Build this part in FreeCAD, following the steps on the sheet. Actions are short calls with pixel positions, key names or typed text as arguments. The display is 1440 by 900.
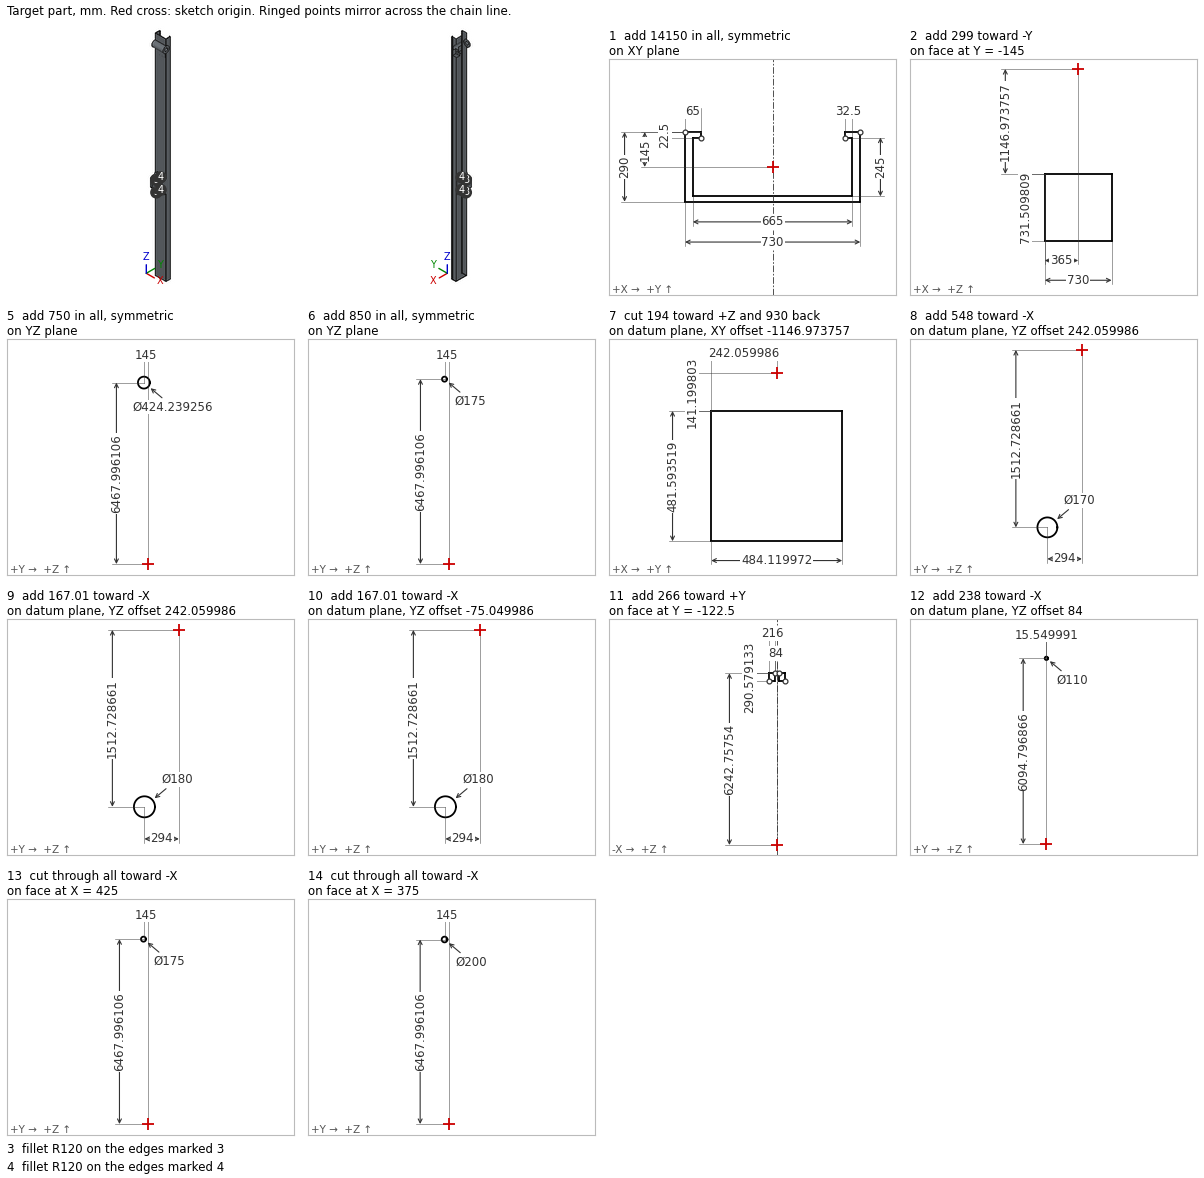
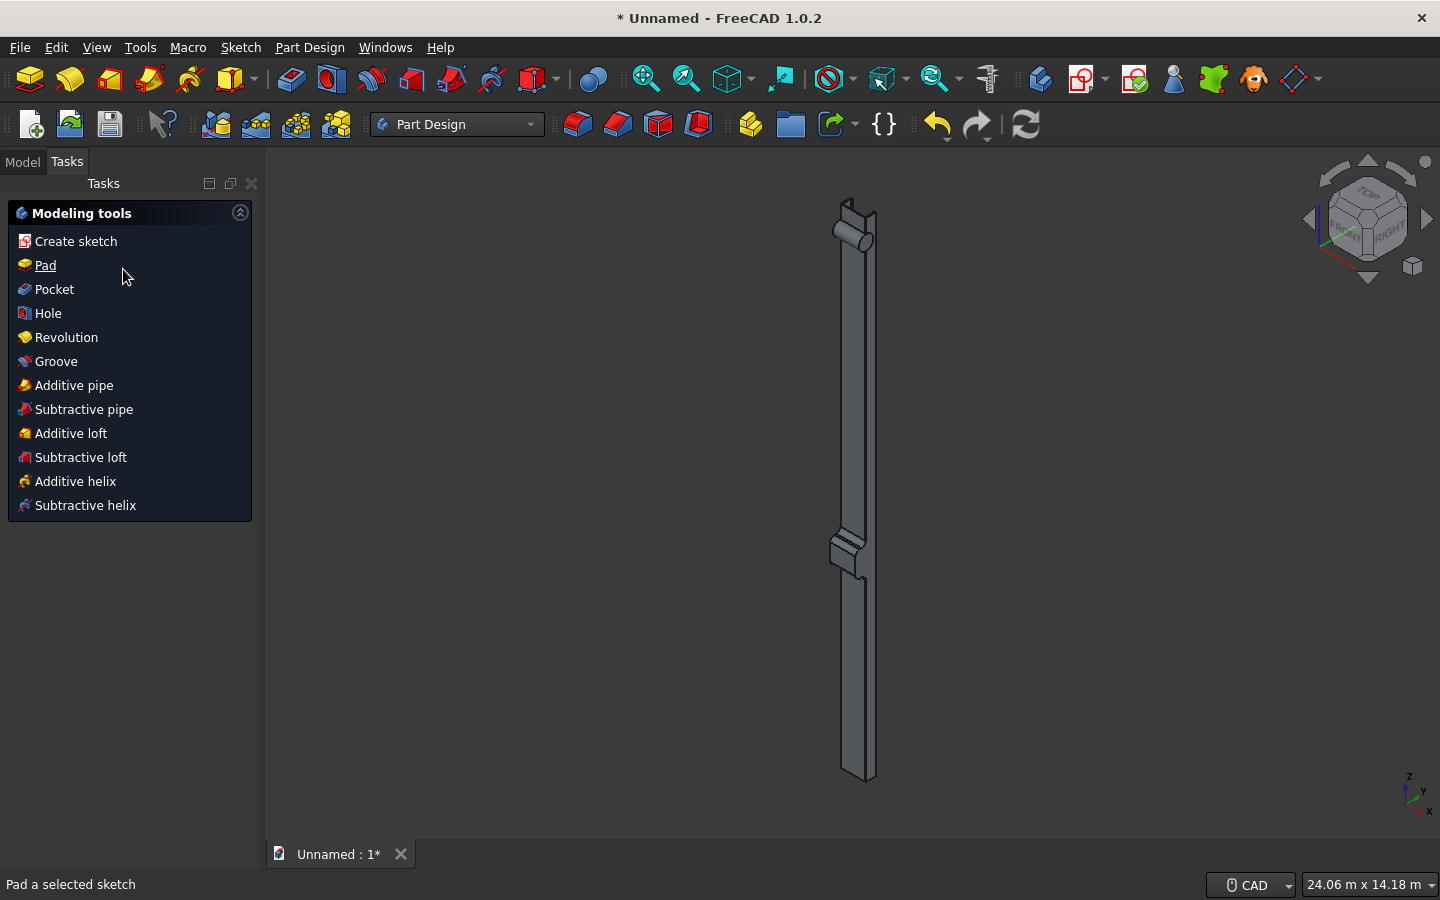
click(30, 80)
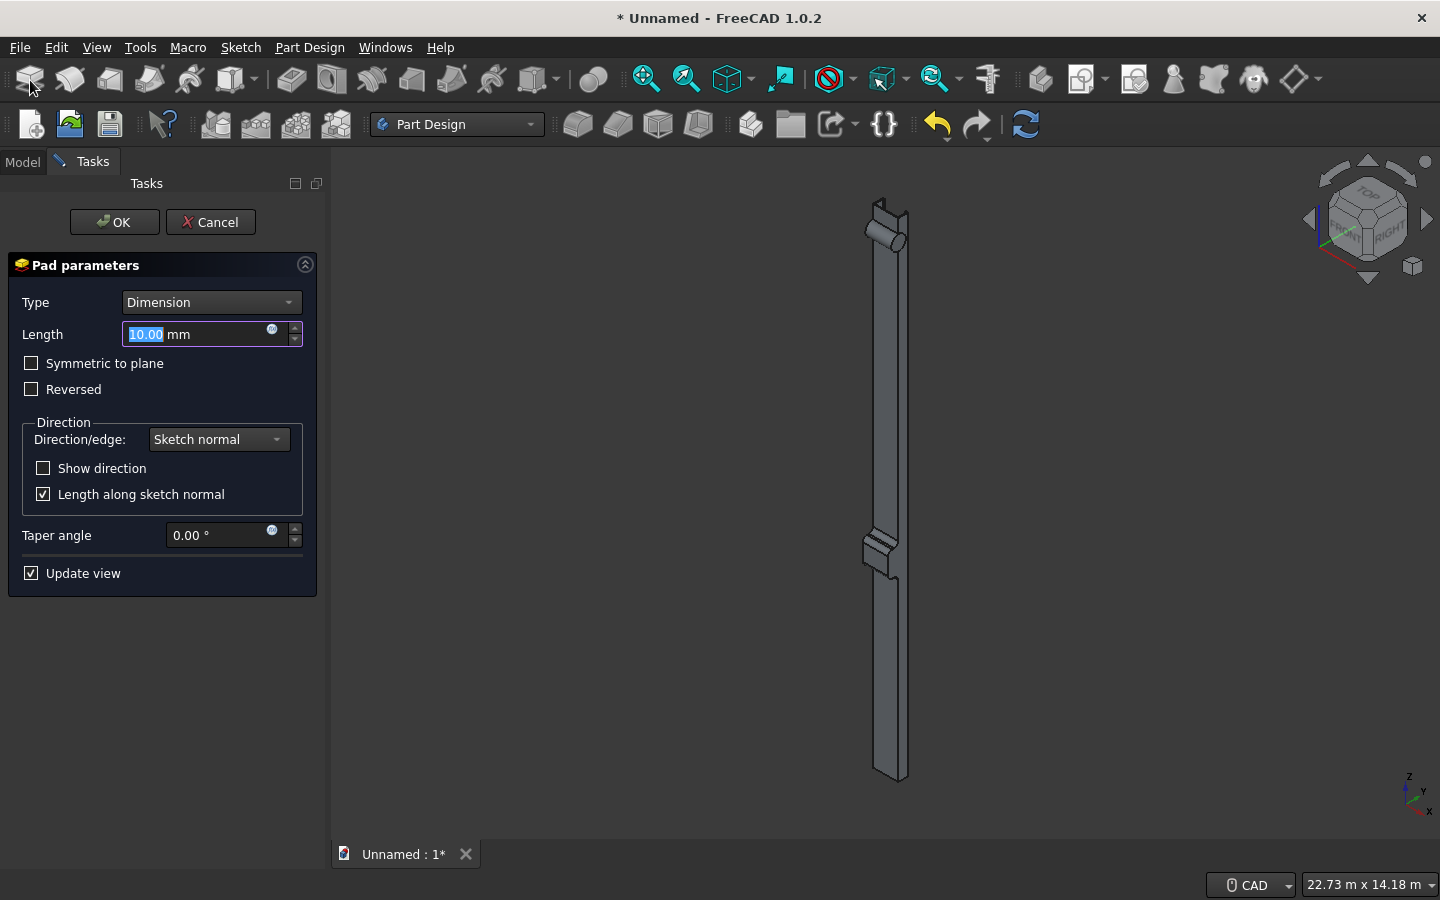
text(850)
key(Tab)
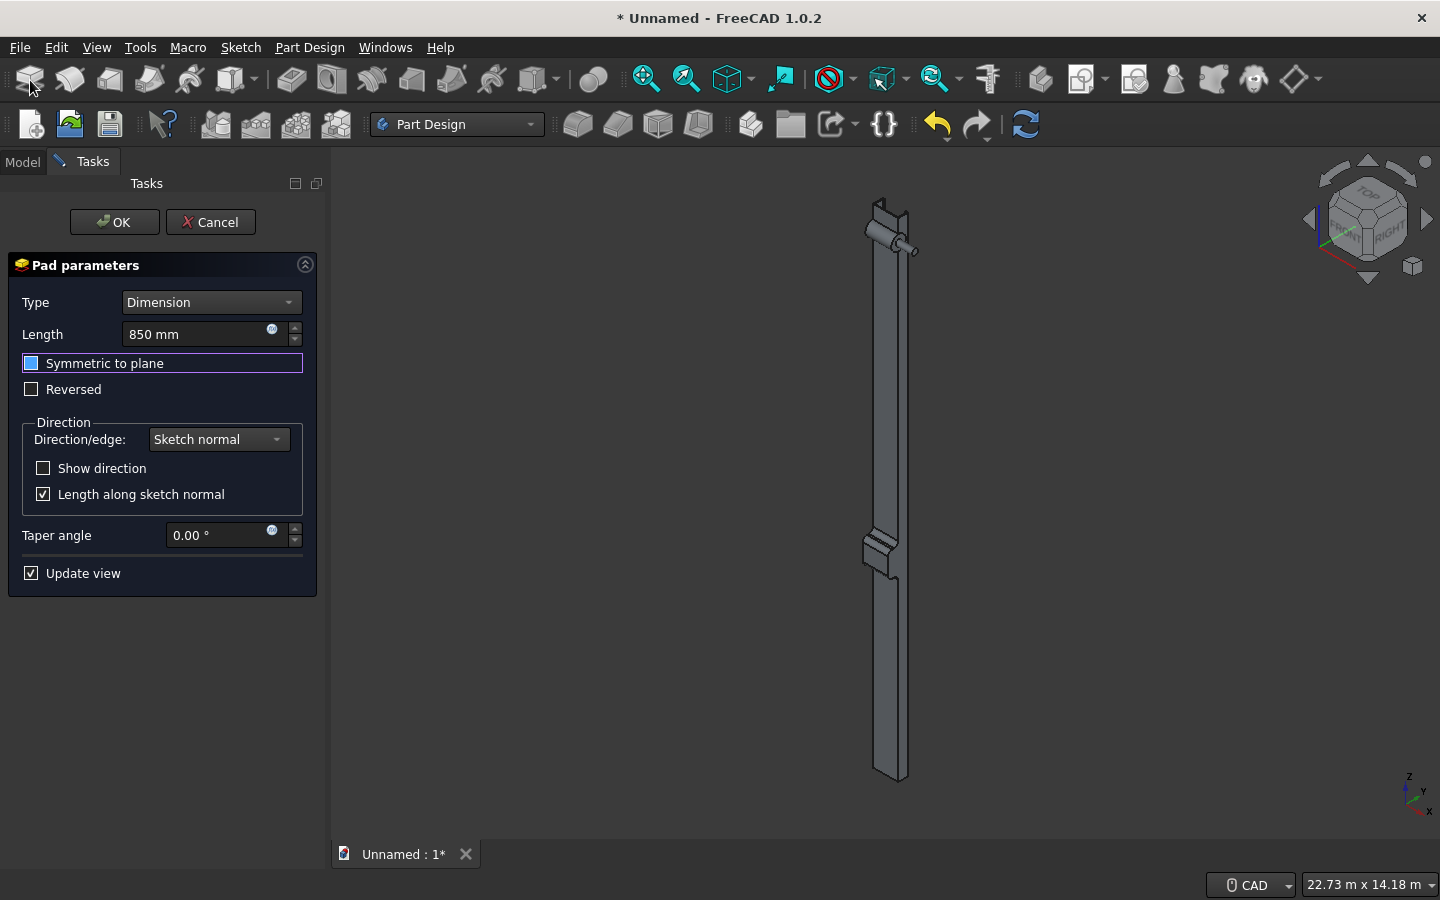
click(30, 363)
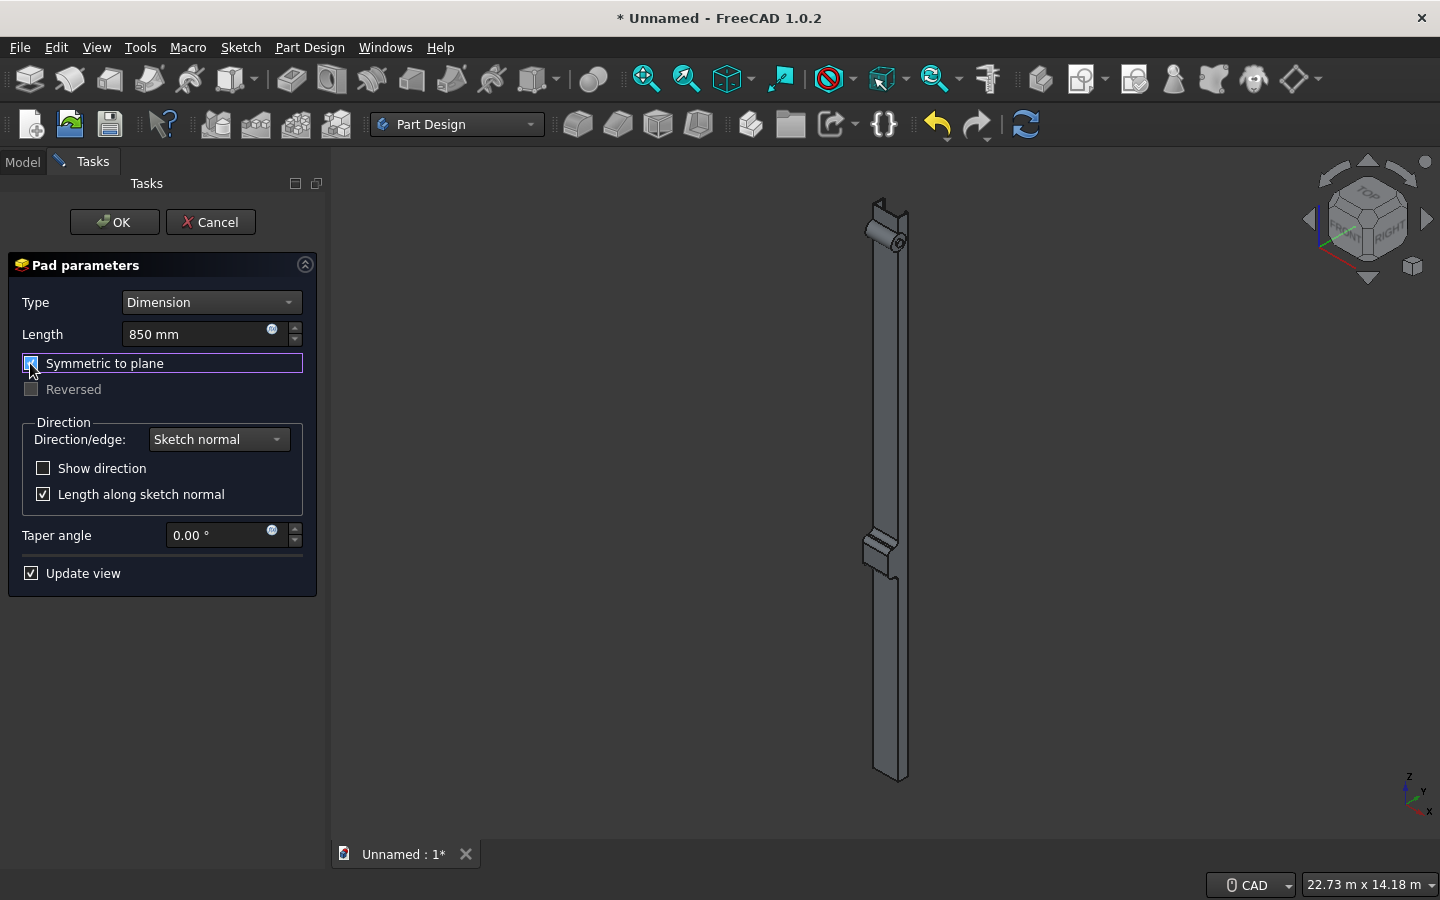
click(115, 222)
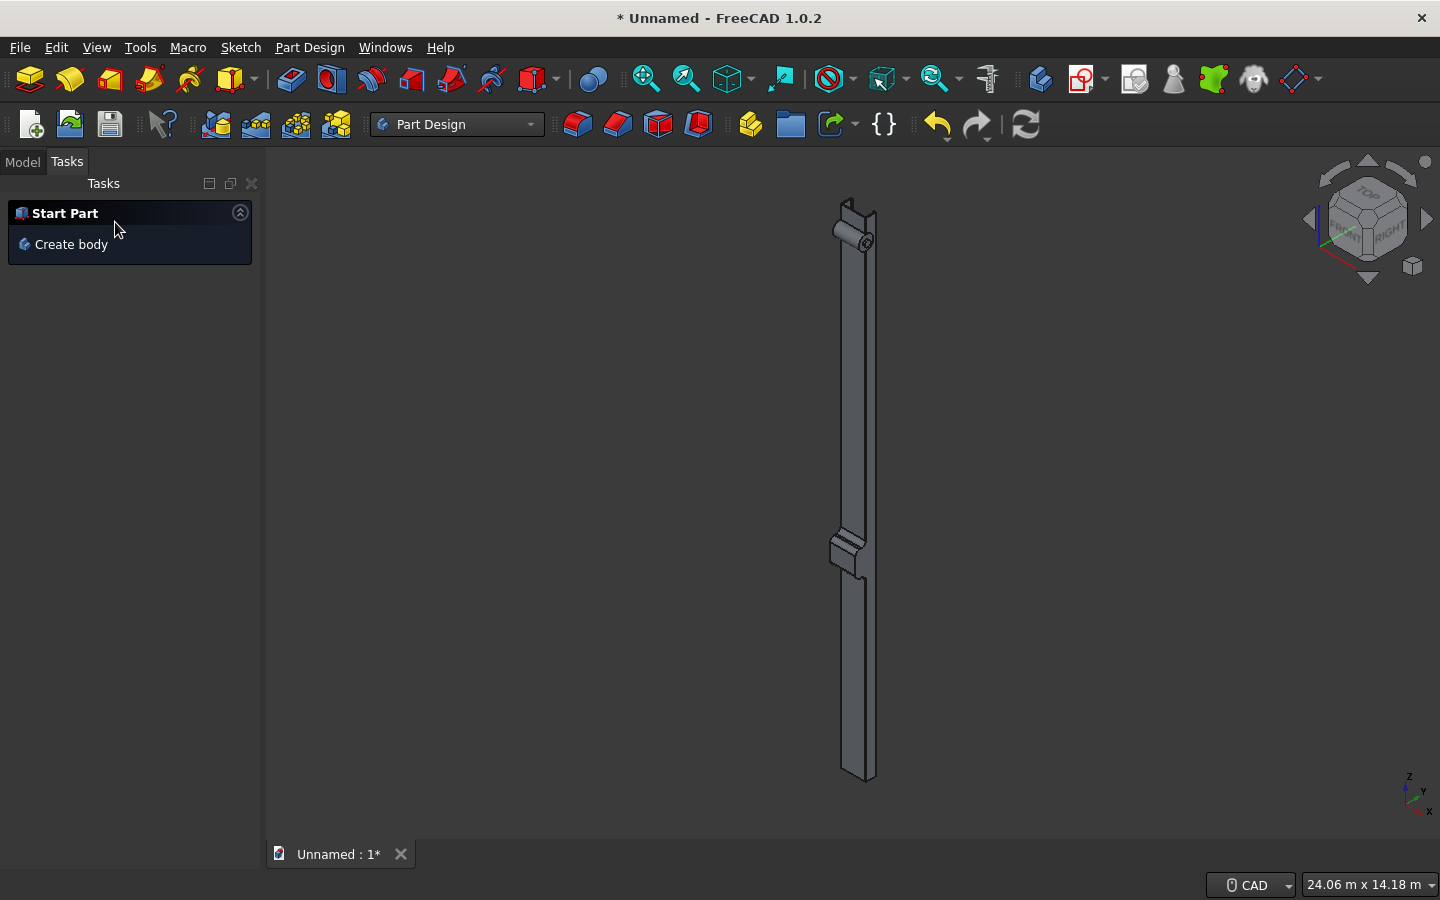
click(23, 161)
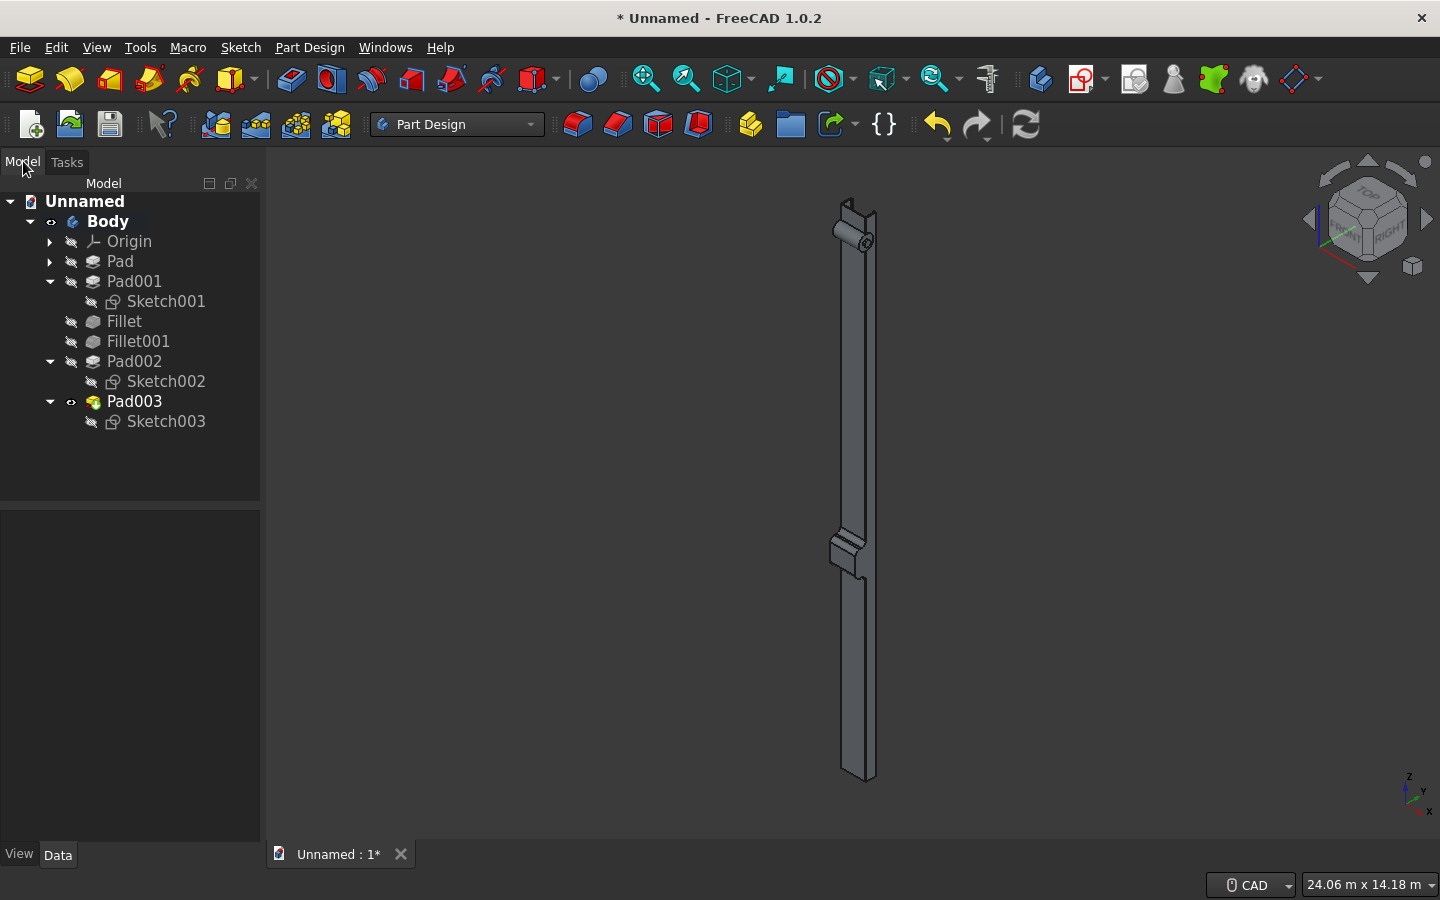
click(50, 242)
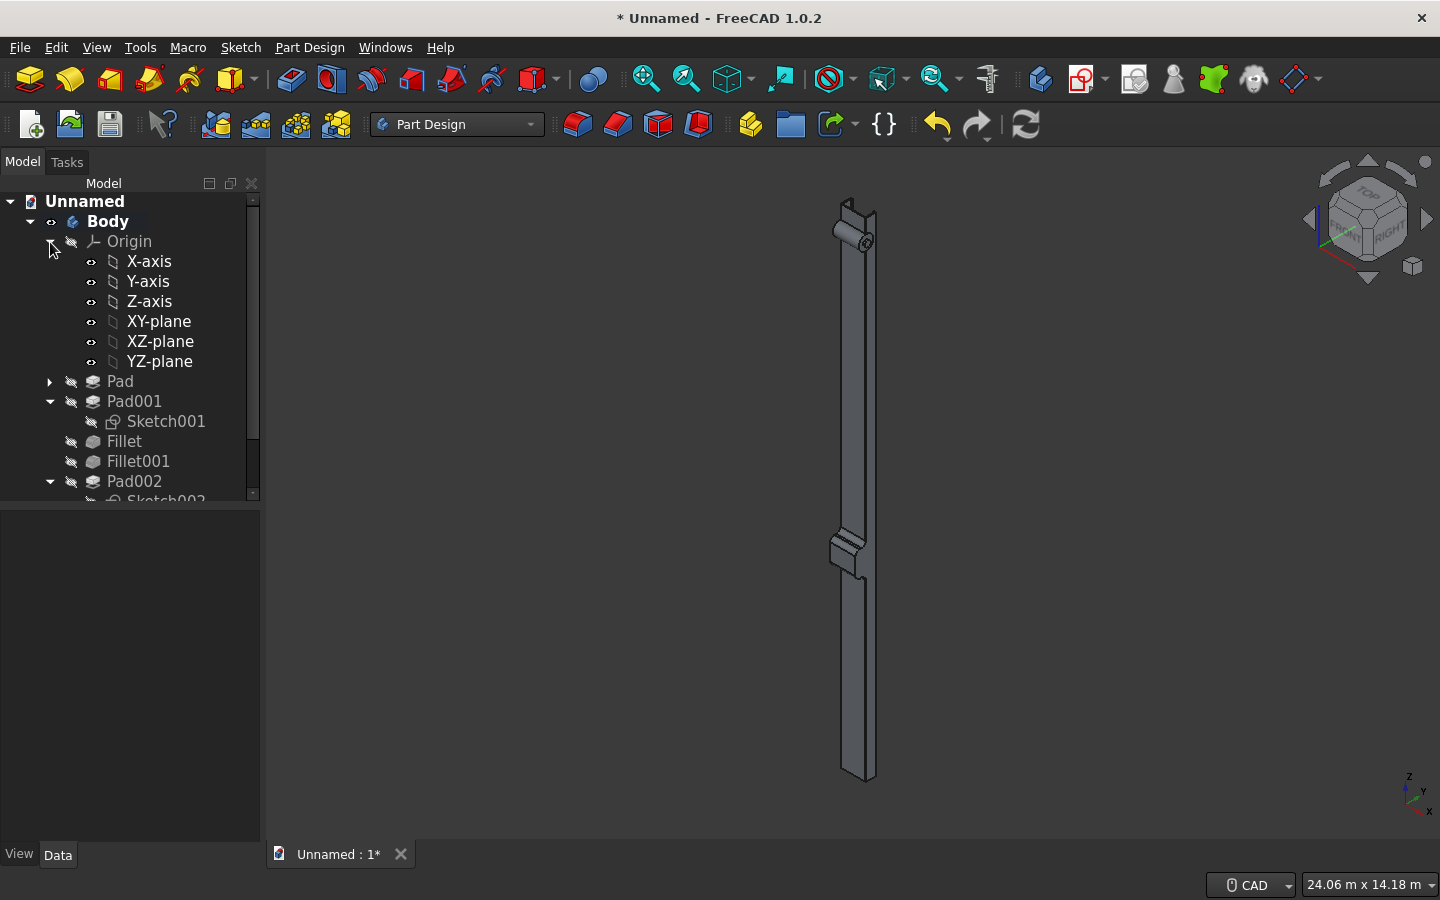
click(136, 322)